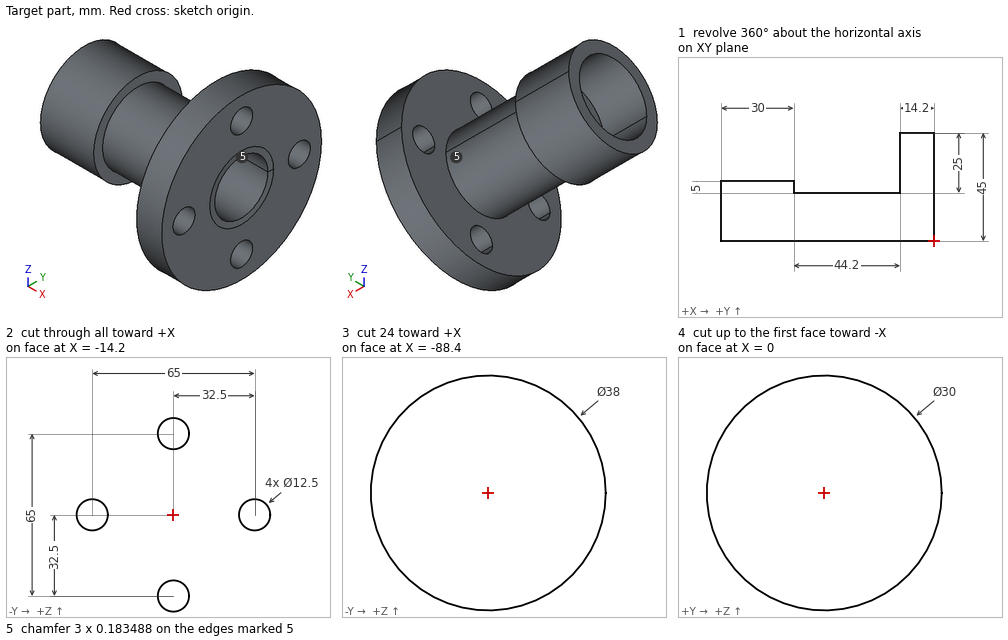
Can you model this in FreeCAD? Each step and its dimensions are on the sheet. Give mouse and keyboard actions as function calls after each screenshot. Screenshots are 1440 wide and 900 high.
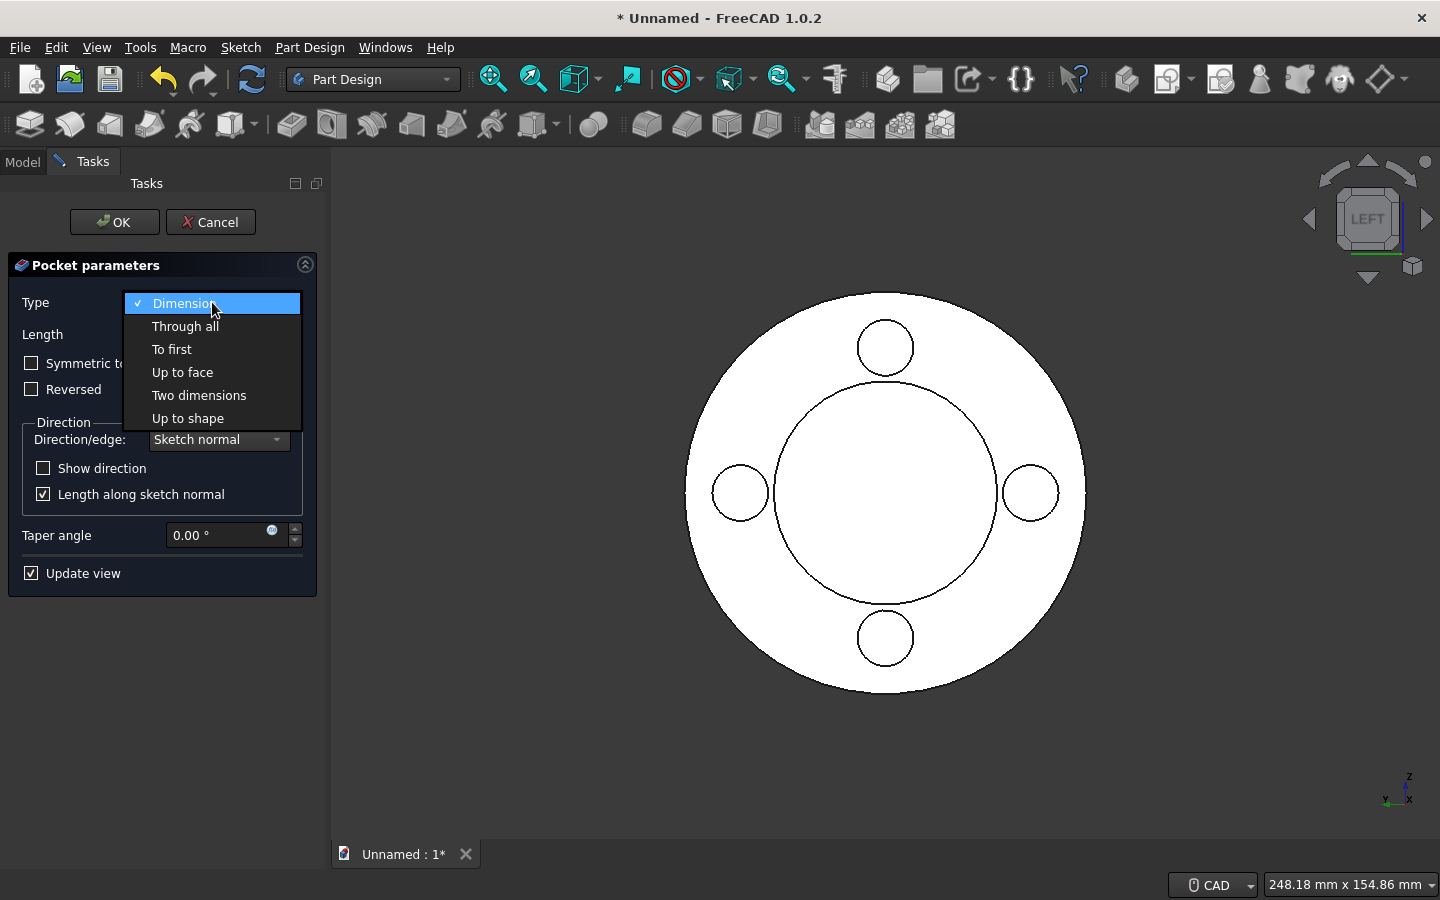
click(212, 326)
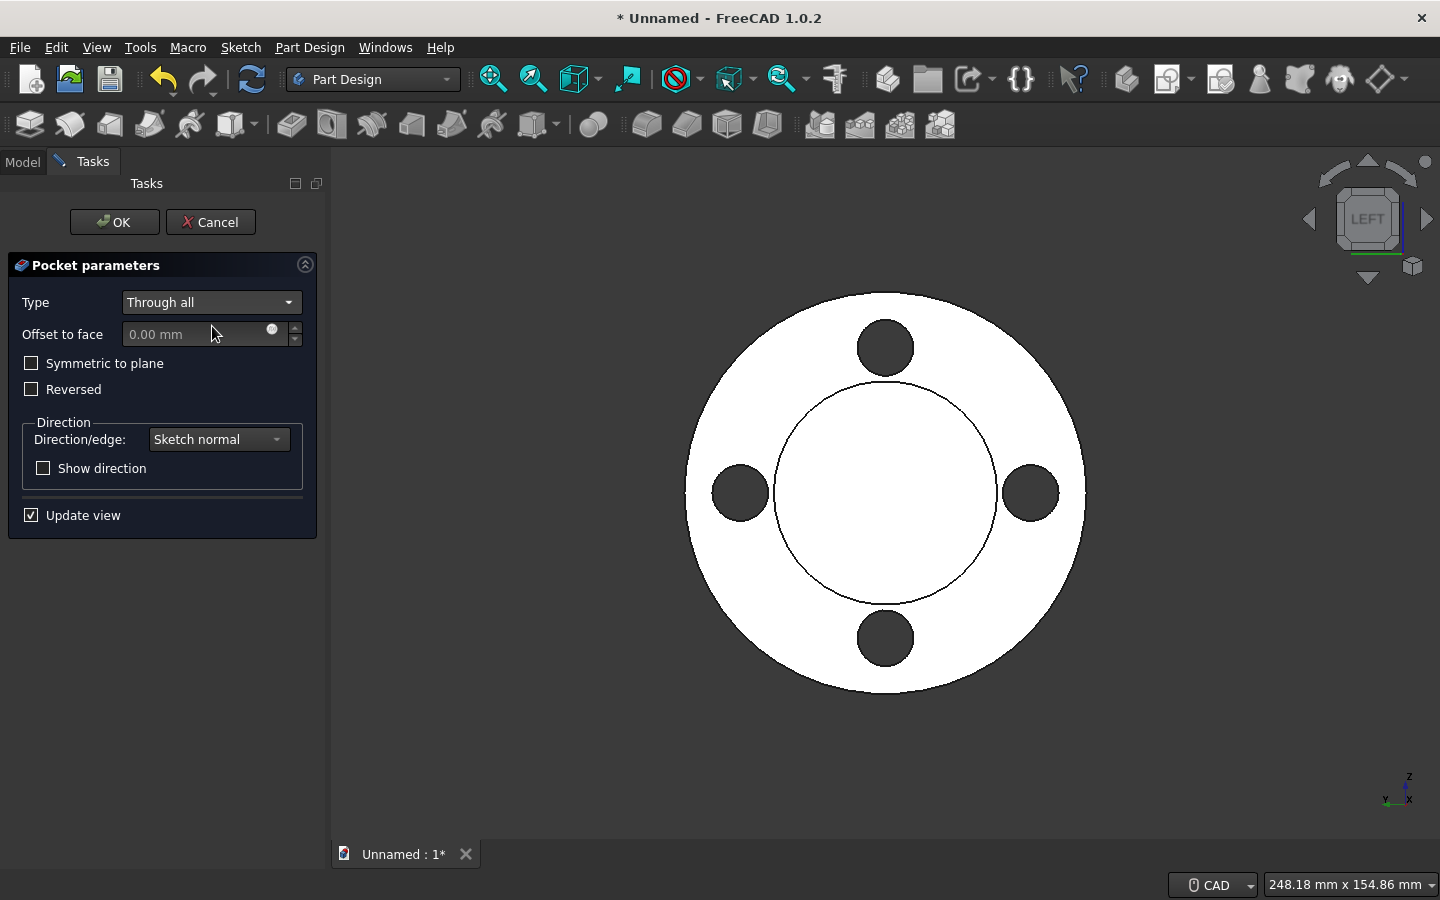
click(115, 222)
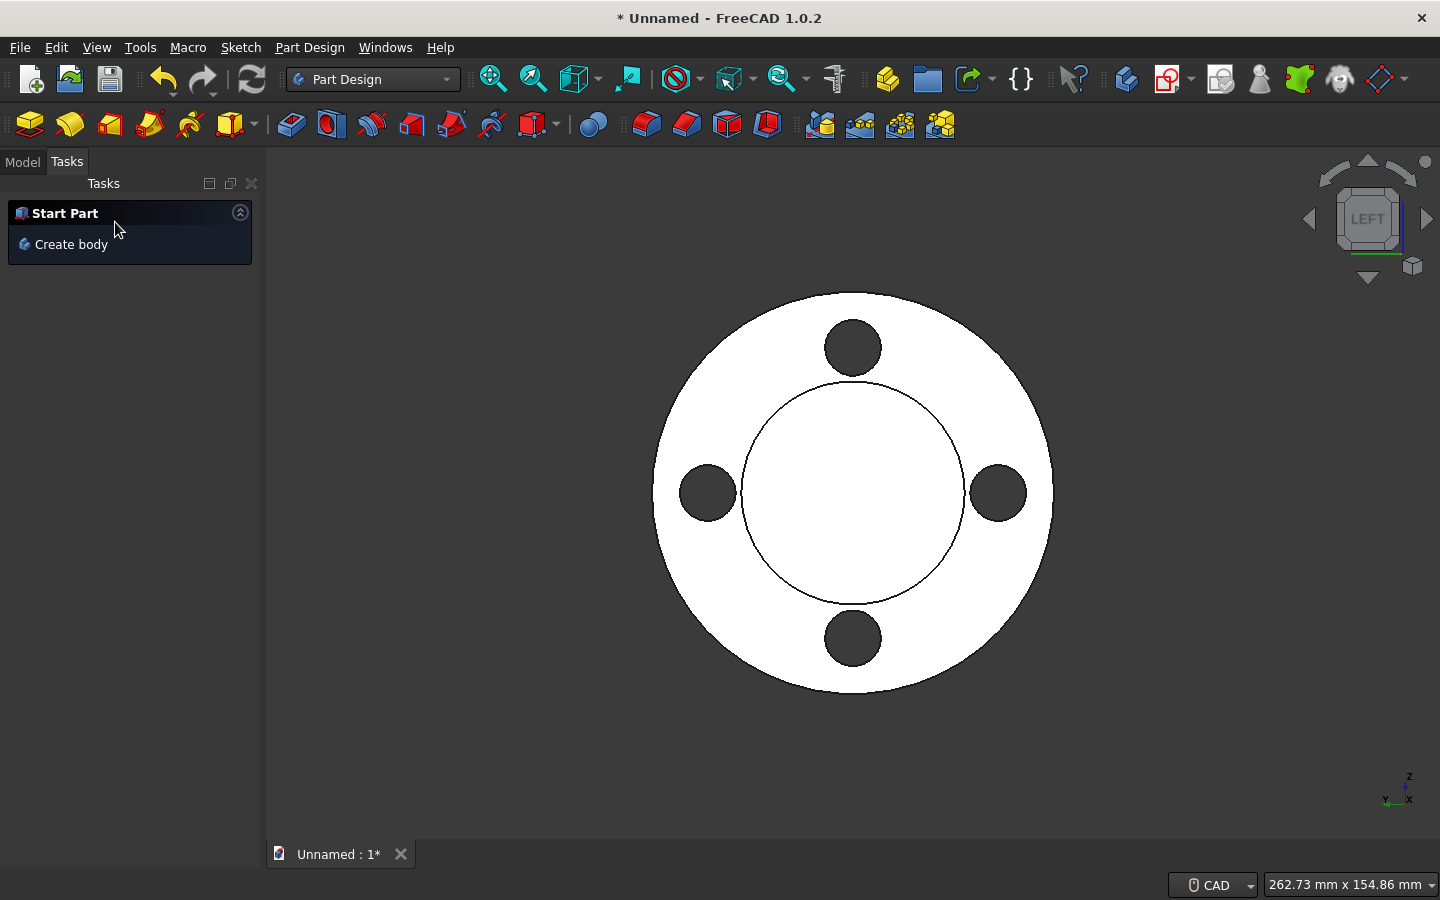
click(853, 492)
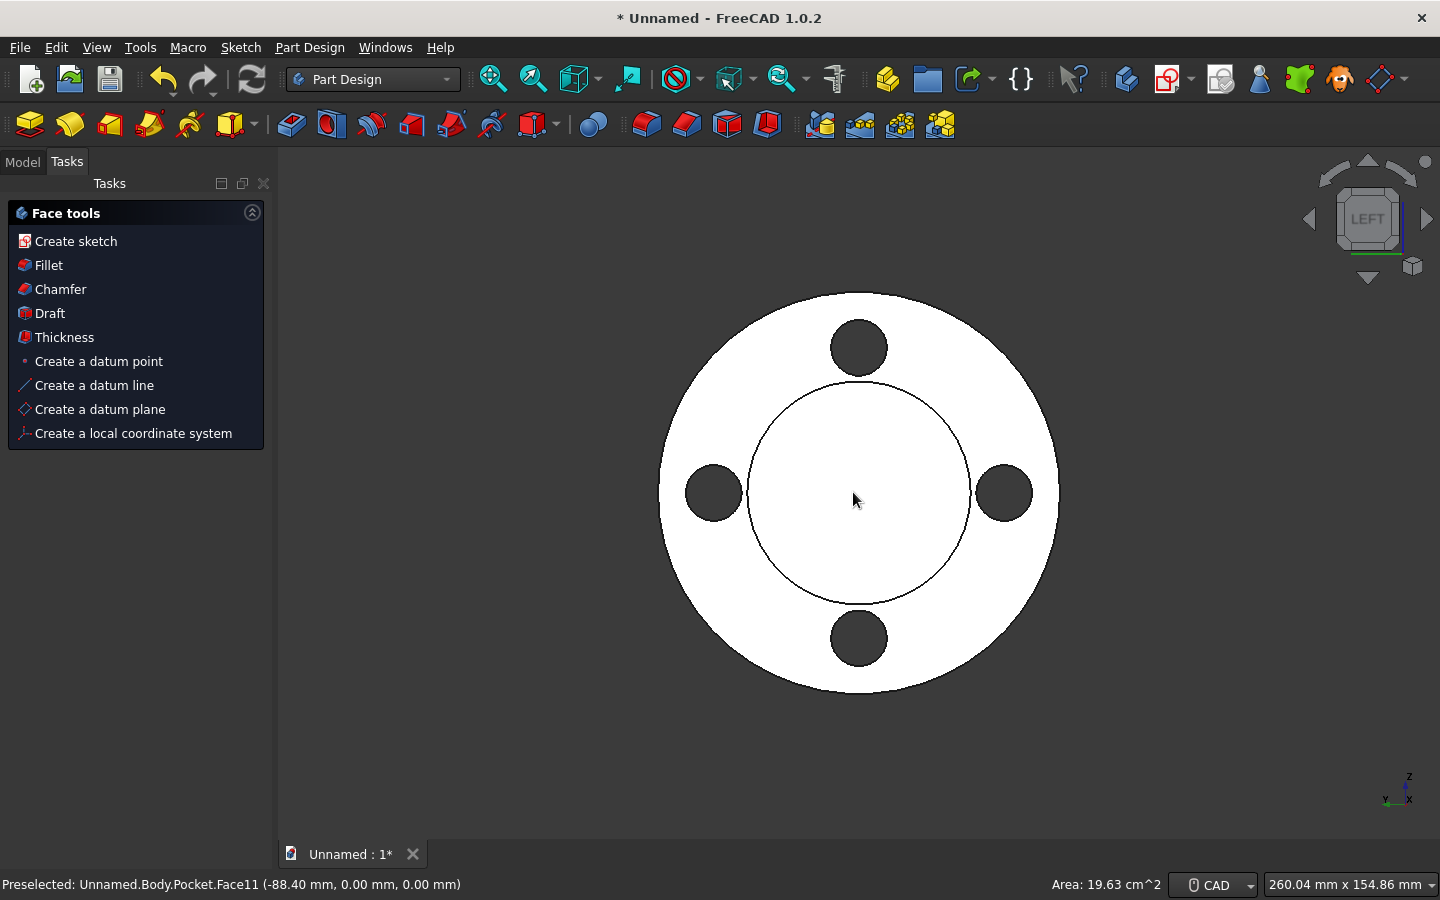
click(1168, 80)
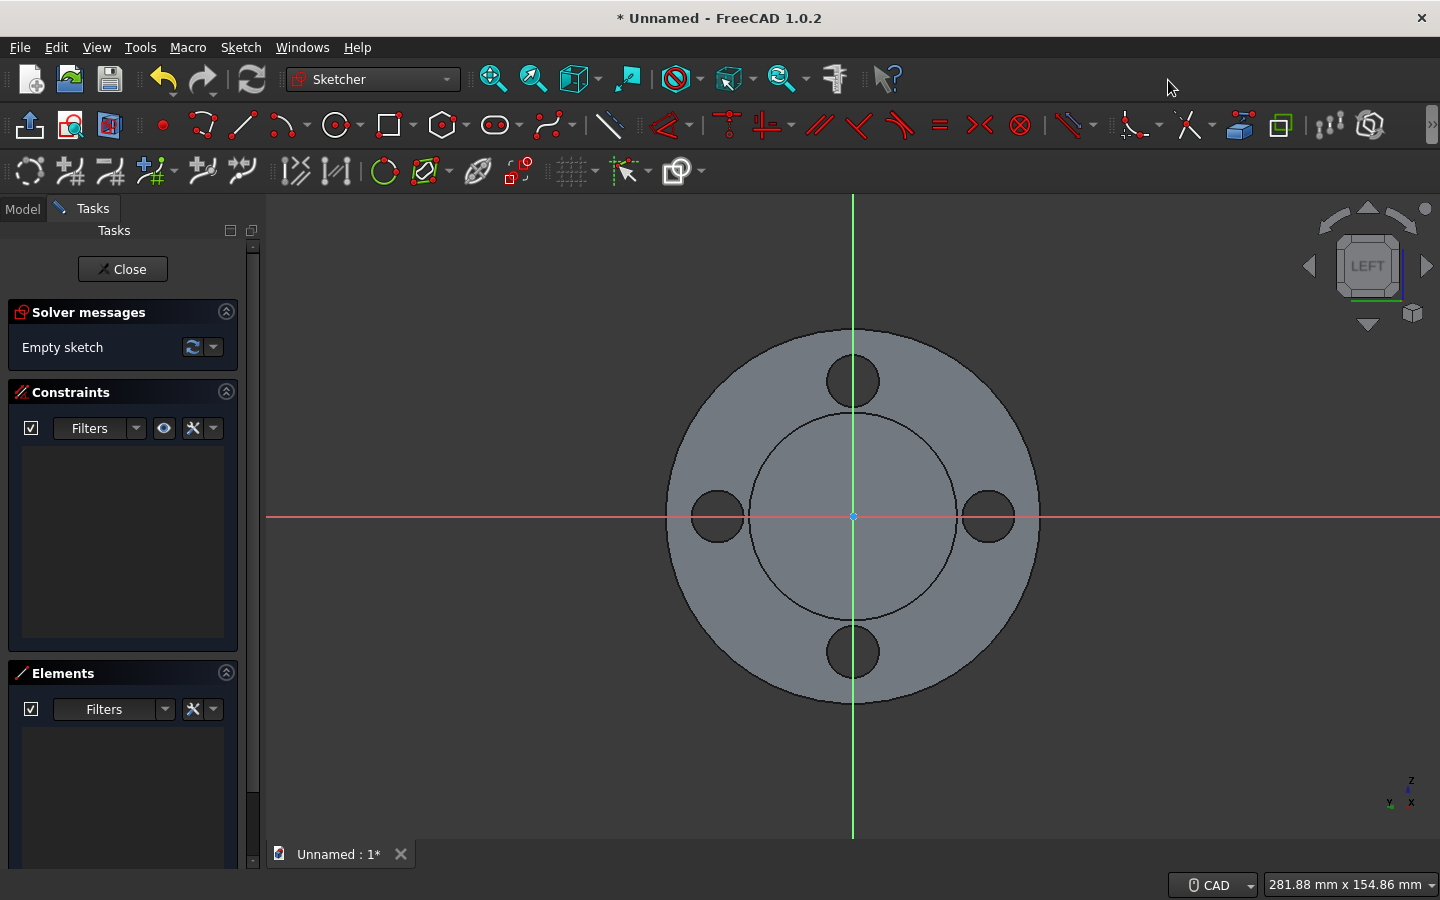
scroll(893, 517, up, 5)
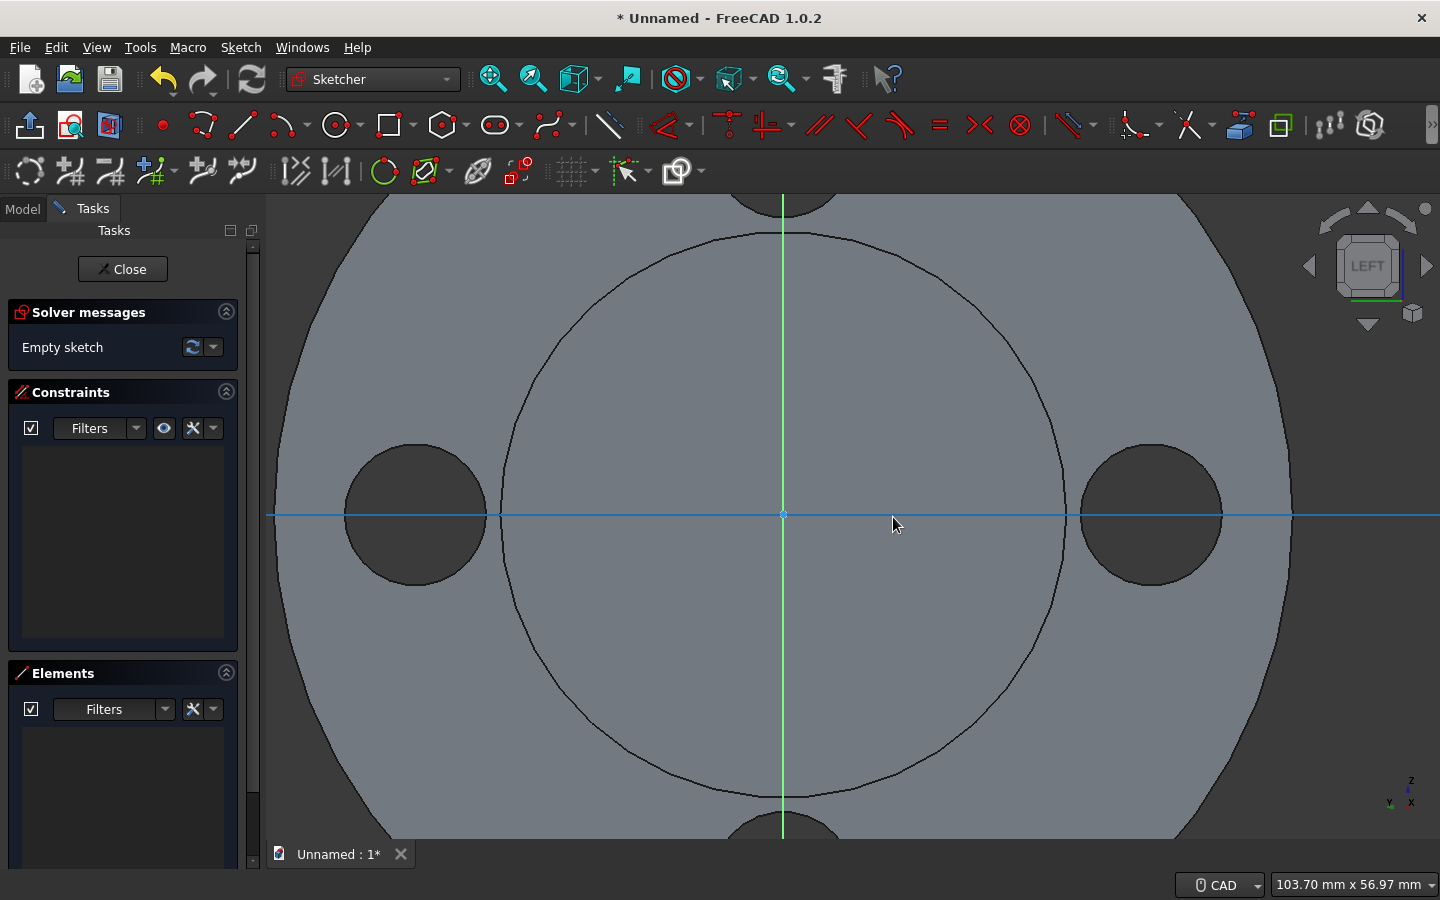
key(g)
key(c)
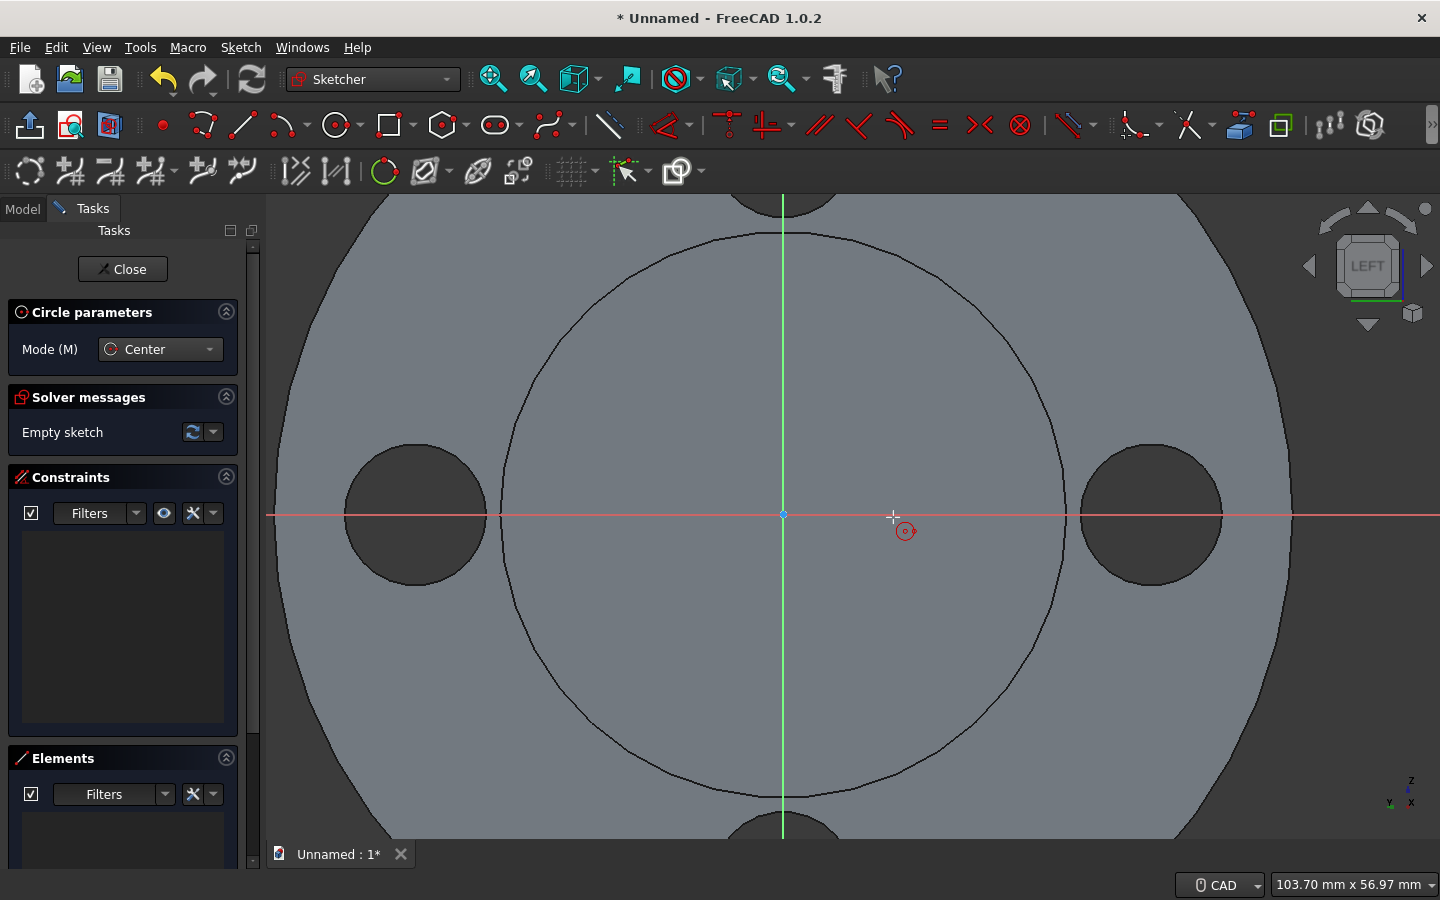
click(783, 515)
click(935, 363)
key(Escape)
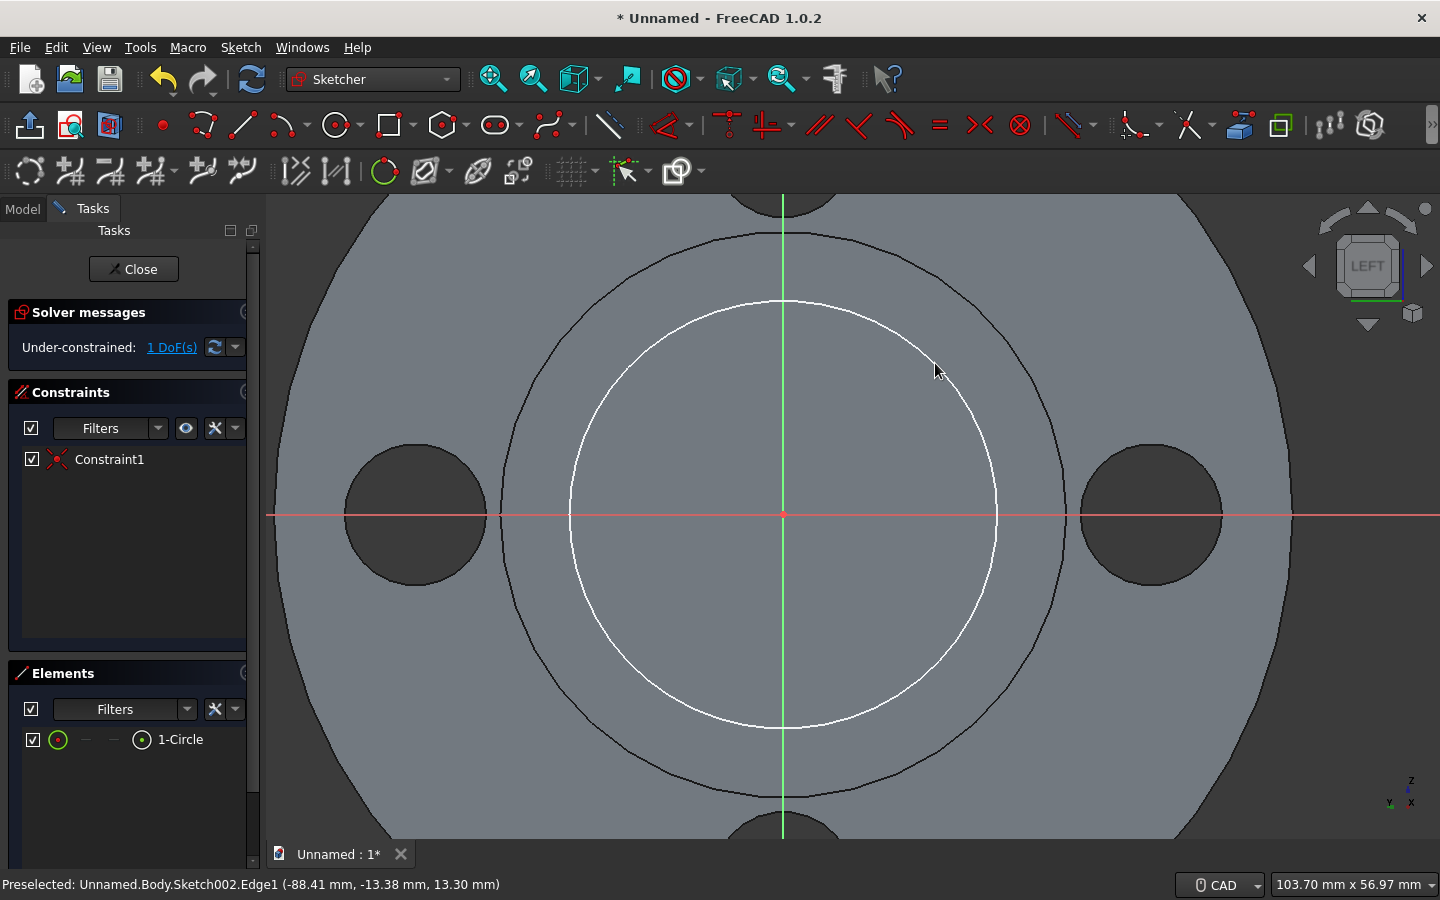
key(d)